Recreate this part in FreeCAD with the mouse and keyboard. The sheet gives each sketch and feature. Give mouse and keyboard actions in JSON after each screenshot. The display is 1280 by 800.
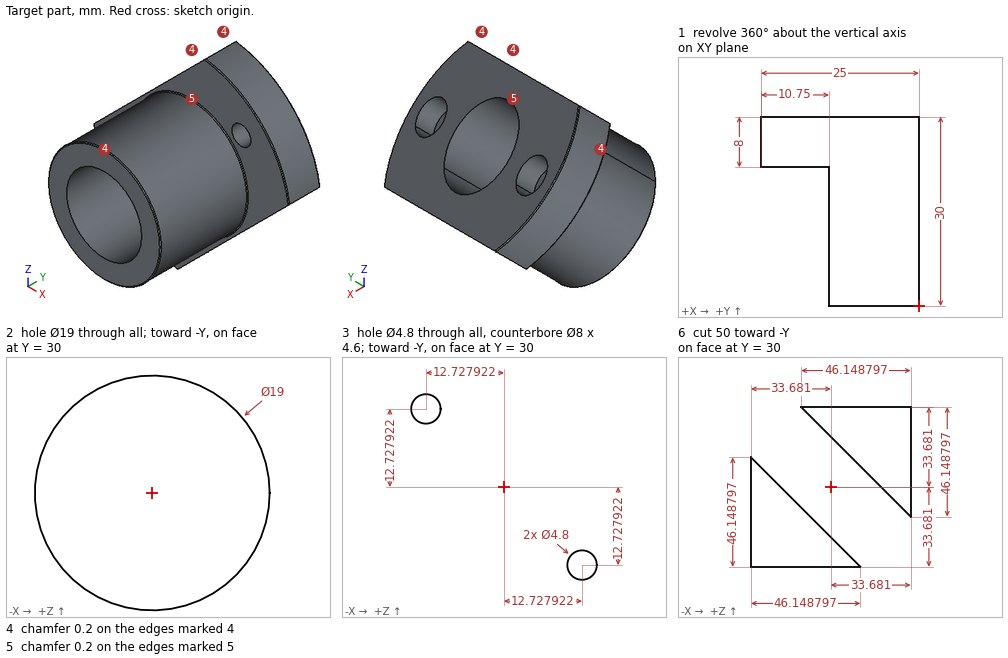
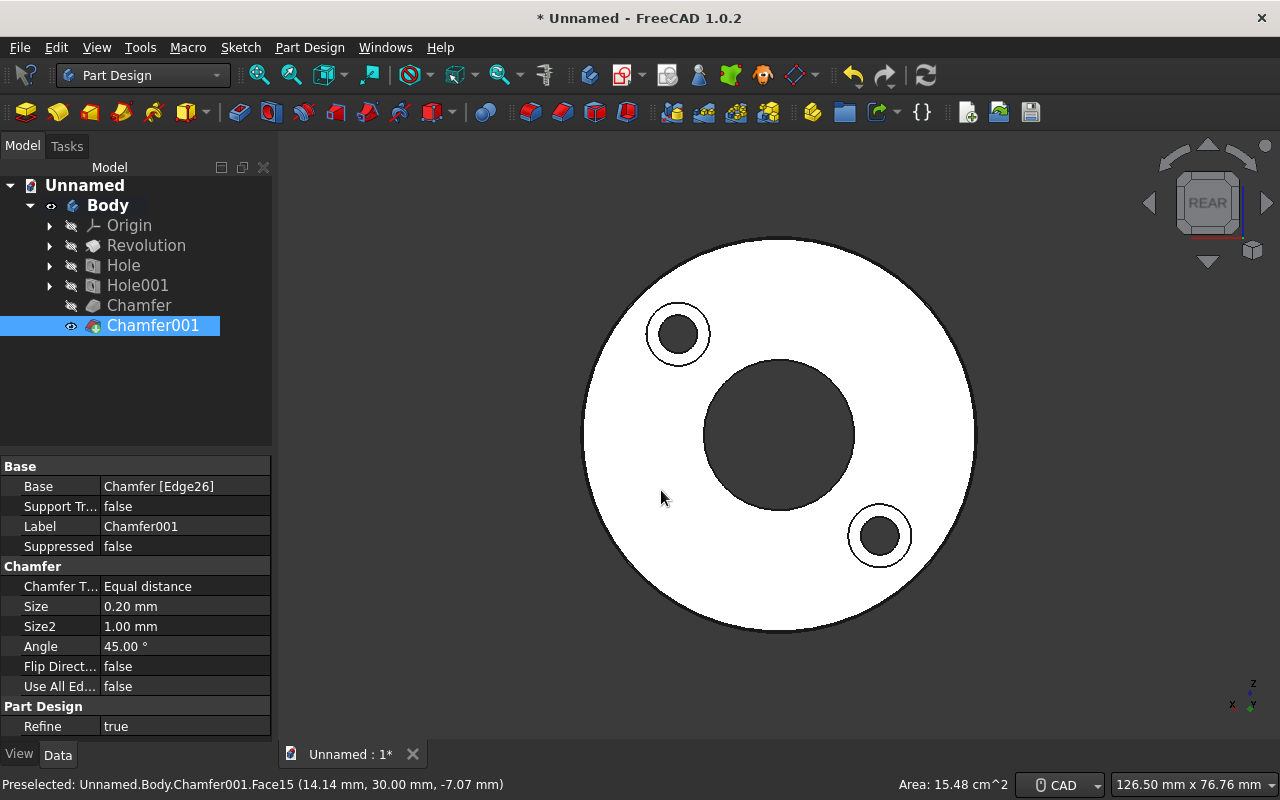
{"action": "left_click", "coordinate": [622, 76]}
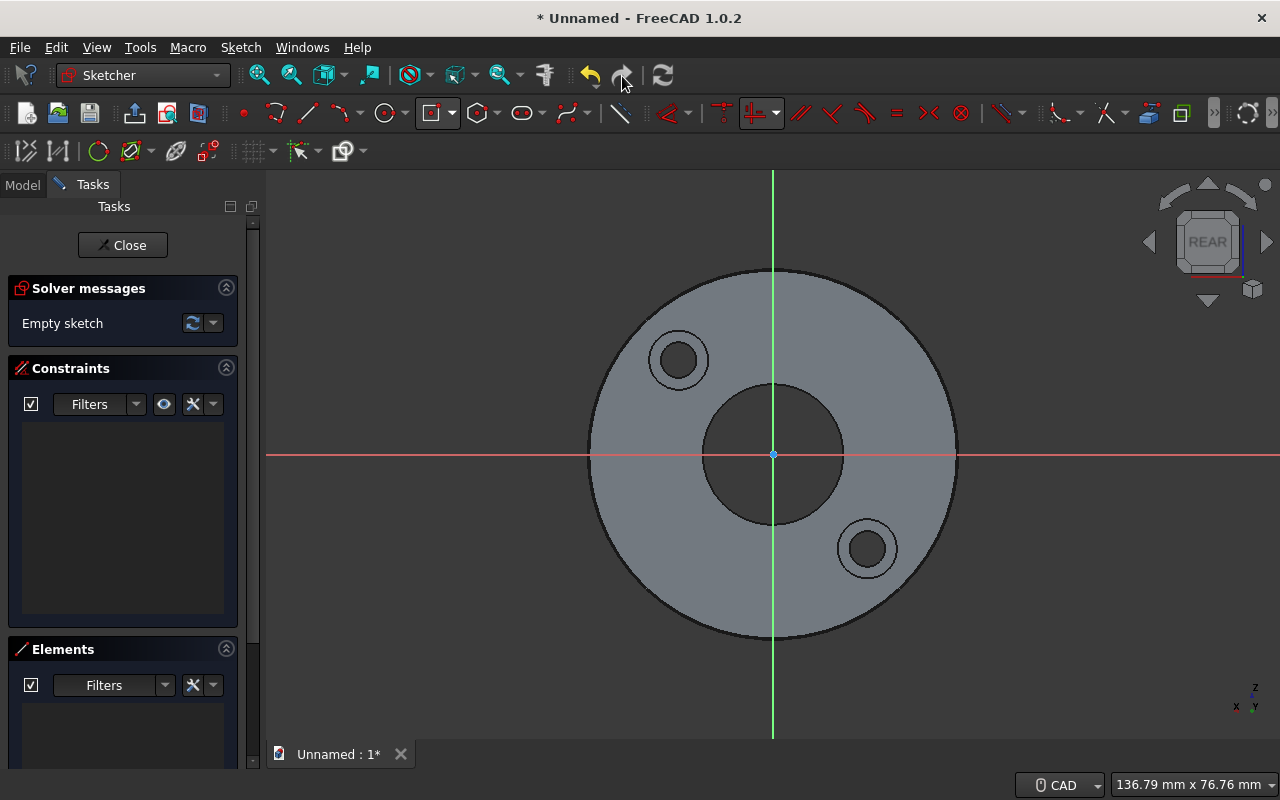
{"action": "scroll", "coordinate": [565, 455], "scroll_direction": "down", "scroll_amount": 2}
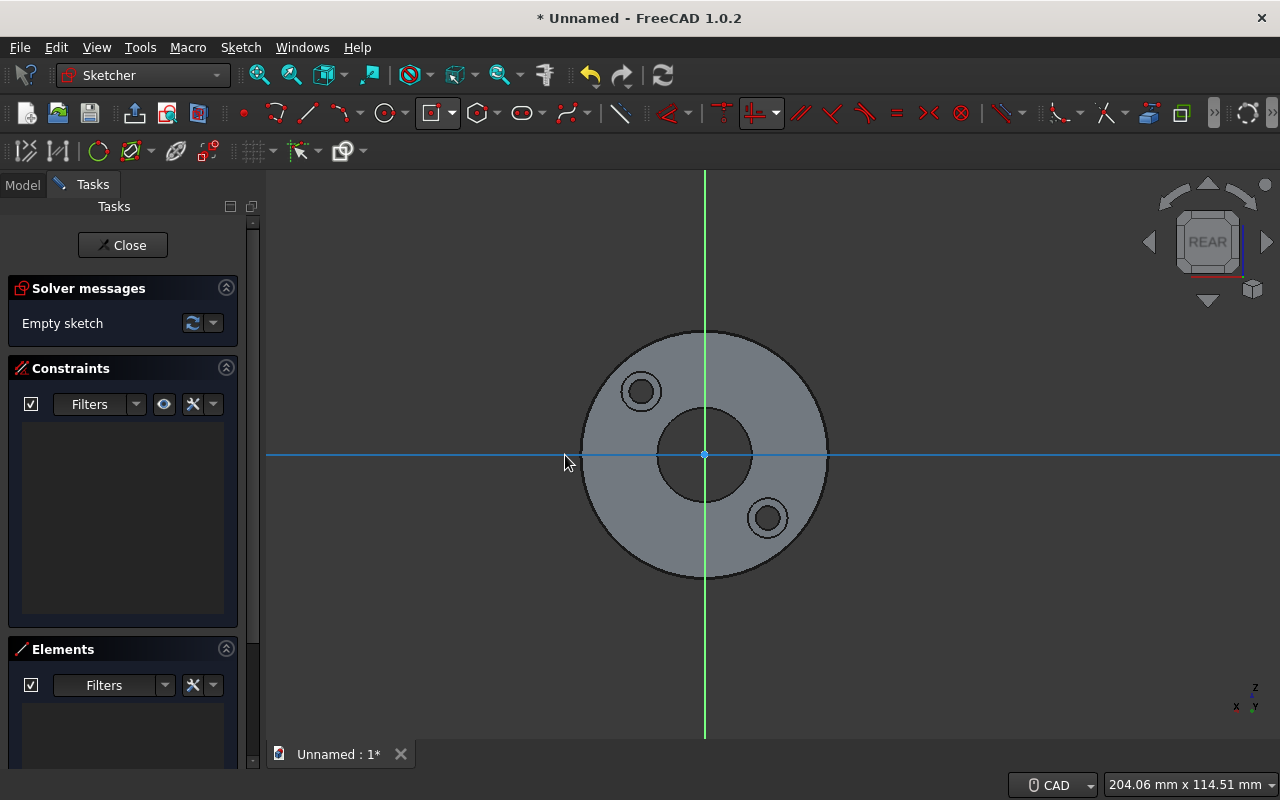
{"action": "left_click", "coordinate": [276, 114]}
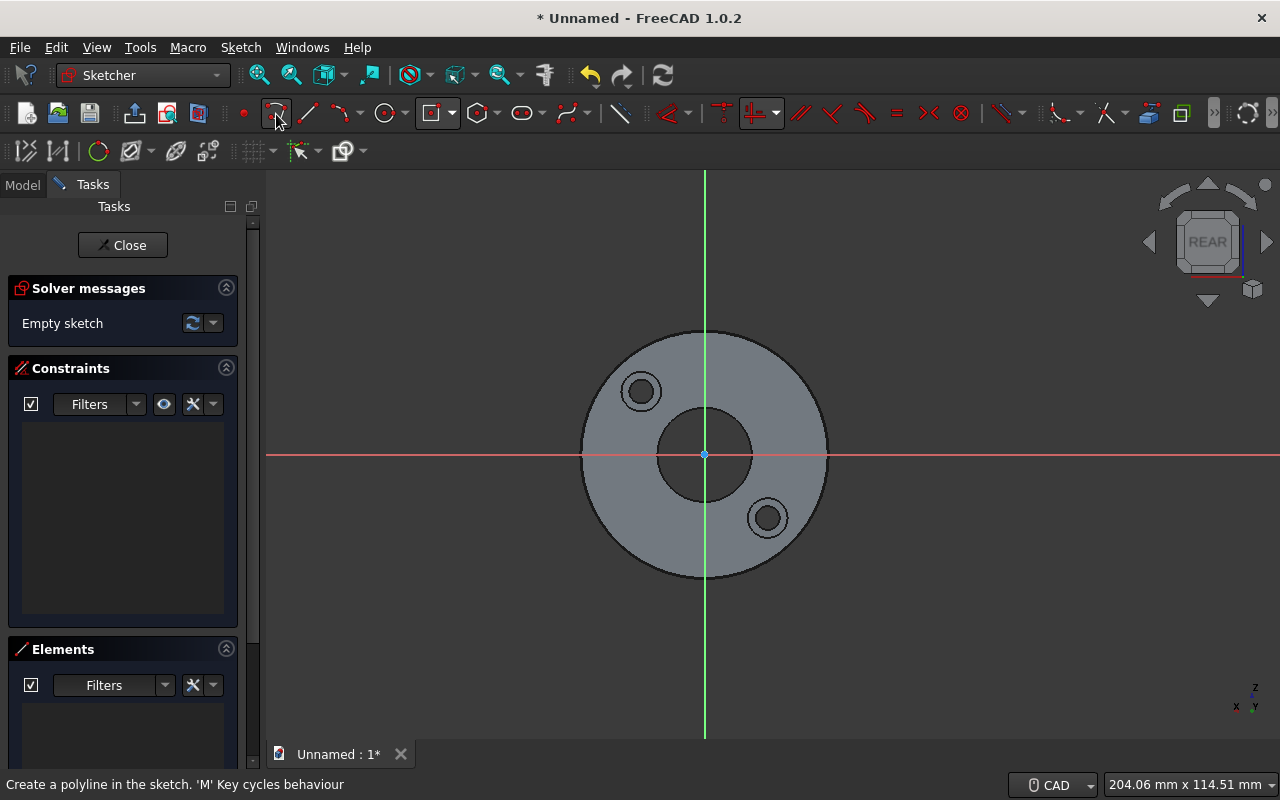
{"action": "left_click", "coordinate": [872, 517]}
{"action": "left_click", "coordinate": [872, 287]}
{"action": "left_click", "coordinate": [643, 287]}
{"action": "left_click", "coordinate": [872, 518]}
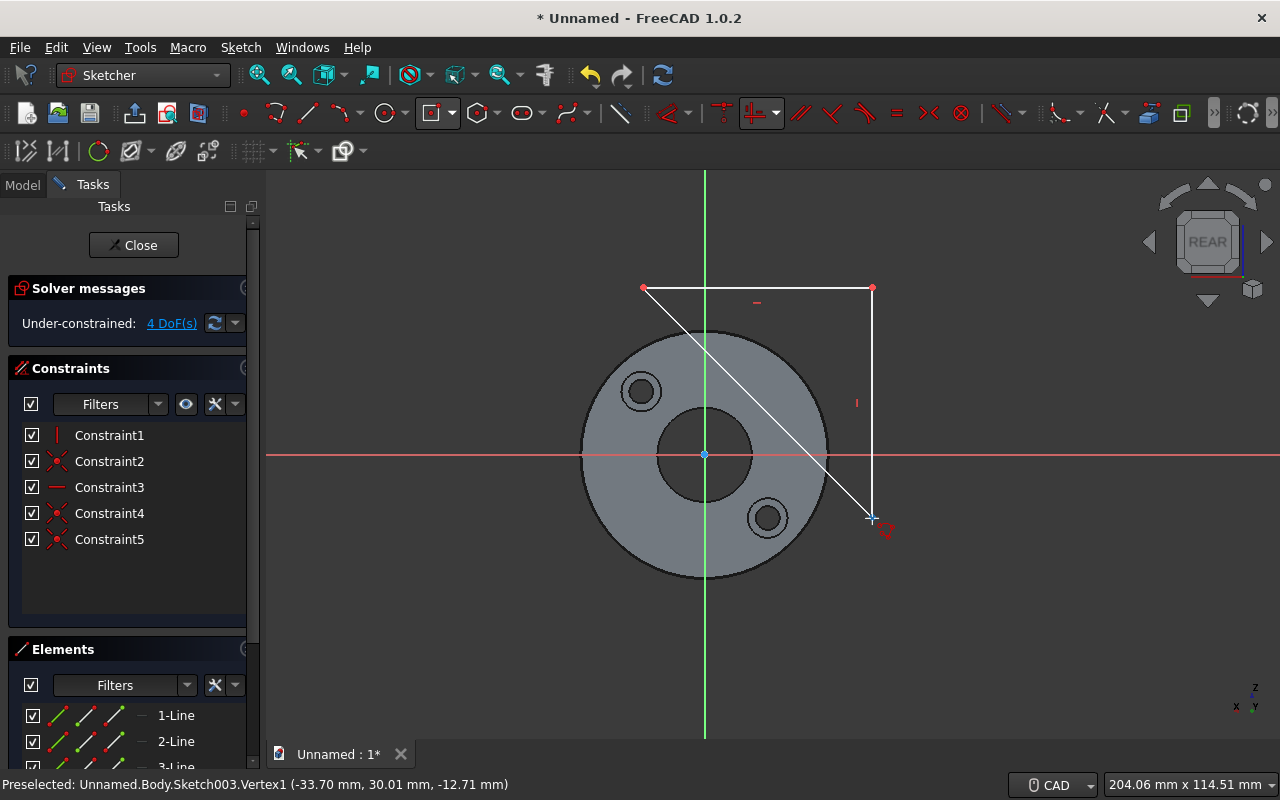
{"action": "left_click", "coordinate": [766, 622]}
{"action": "left_click", "coordinate": [537, 393]}
{"action": "left_click", "coordinate": [537, 622]}
{"action": "left_click", "coordinate": [766, 623]}
{"action": "key", "text": "Escape"}
{"action": "key", "text": "Escape"}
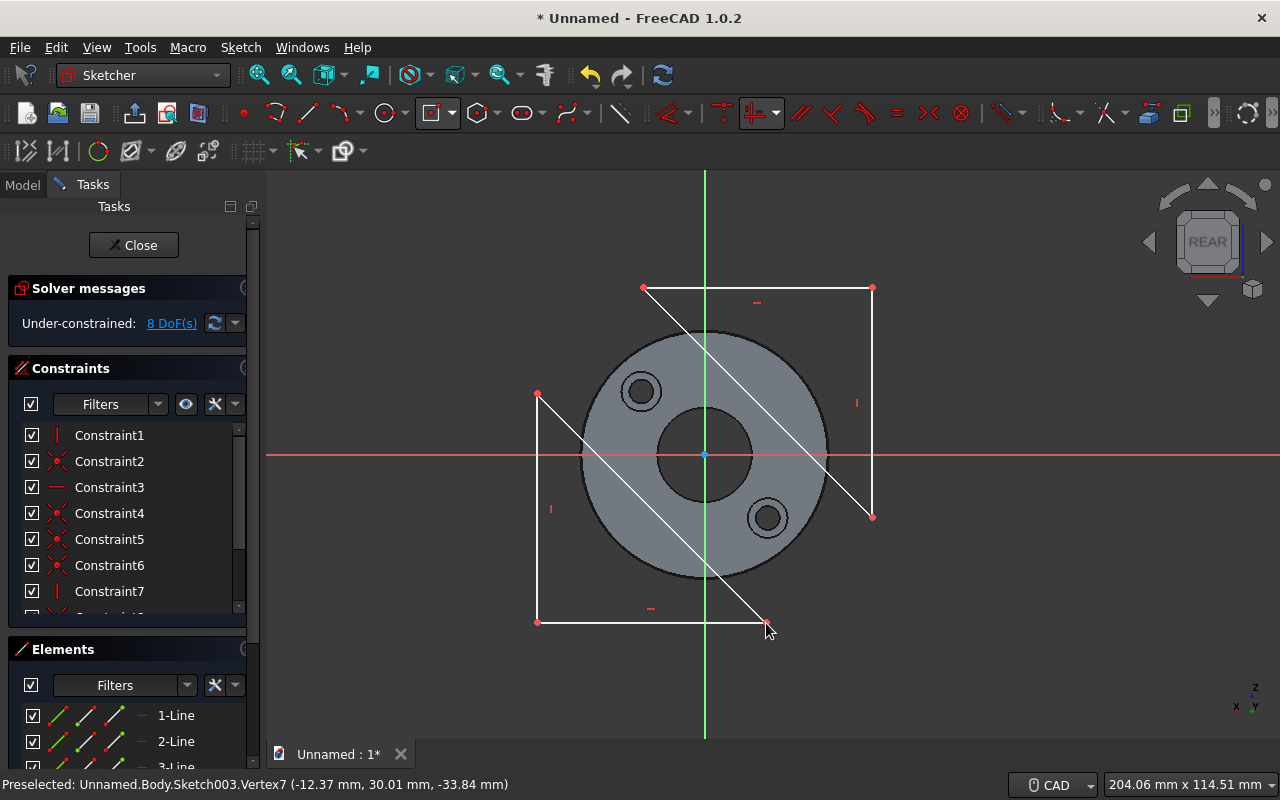
{"action": "left_click", "coordinate": [668, 114]}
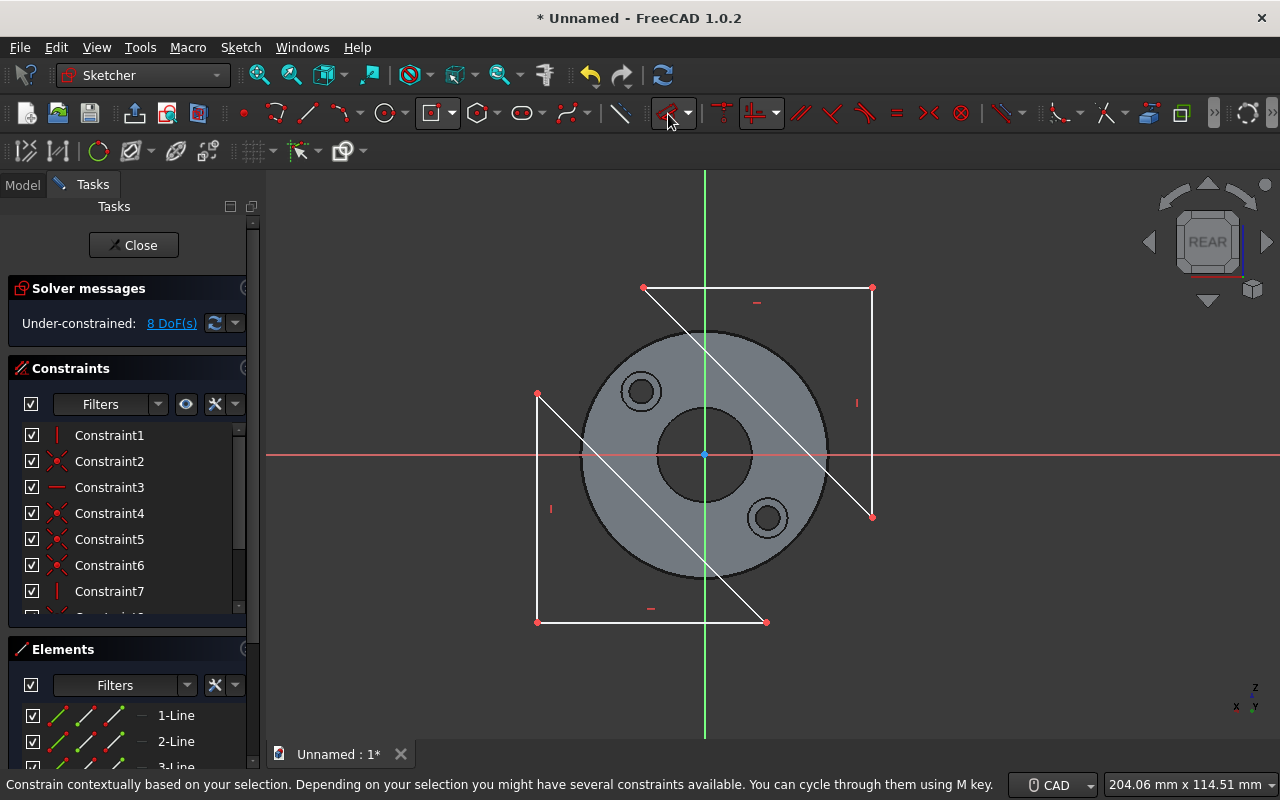
{"action": "left_click", "coordinate": [872, 518]}
{"action": "left_click", "coordinate": [788, 552]}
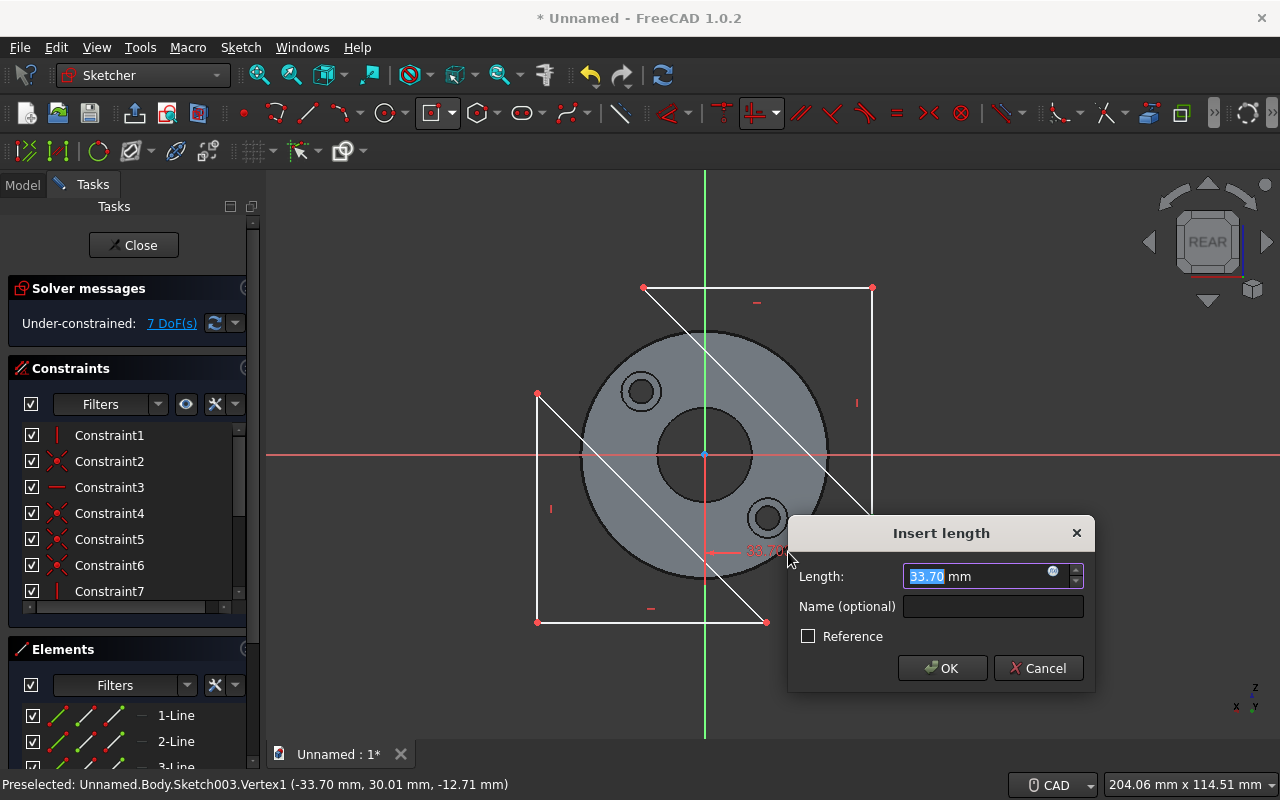
{"action": "type", "text": "33.681"}
{"action": "key", "text": "Return"}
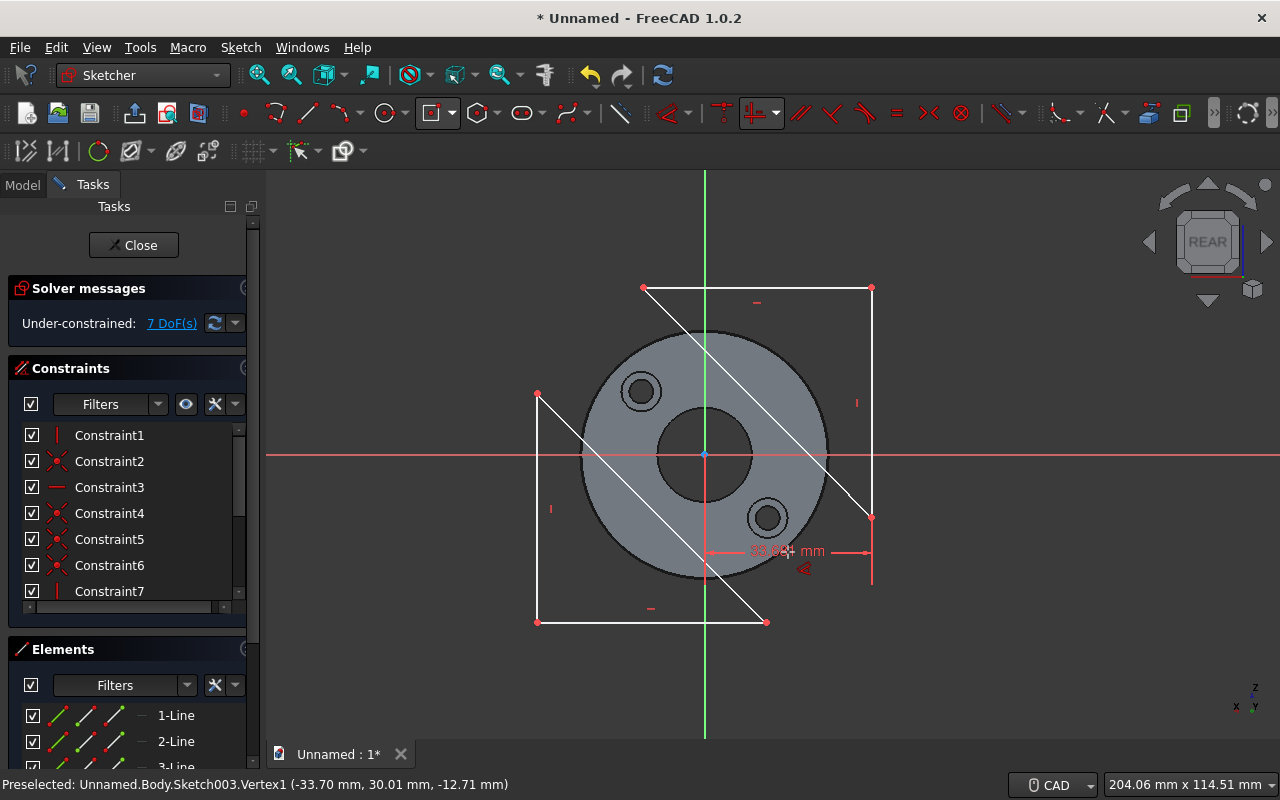
{"action": "left_click", "coordinate": [872, 288]}
{"action": "left_click", "coordinate": [906, 371]}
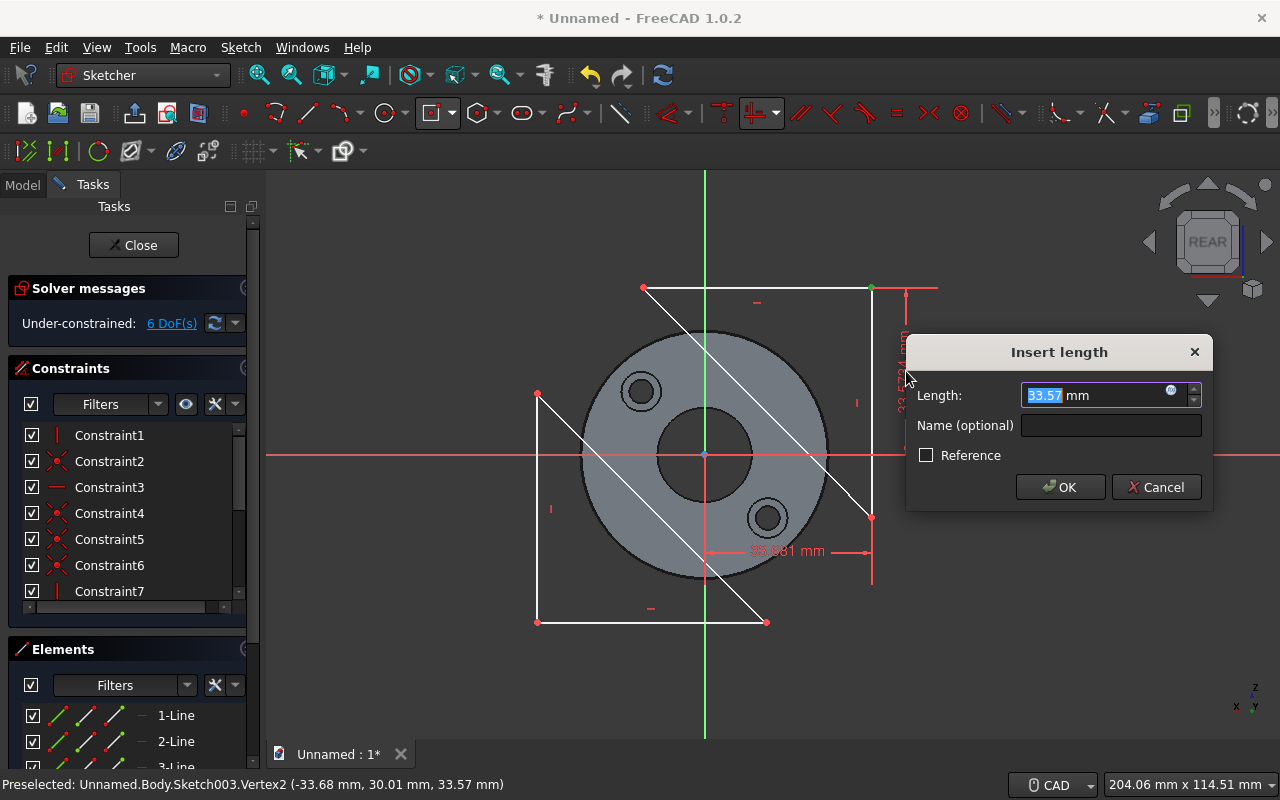
{"action": "type", "text": "33.681"}
{"action": "key", "text": "Return"}